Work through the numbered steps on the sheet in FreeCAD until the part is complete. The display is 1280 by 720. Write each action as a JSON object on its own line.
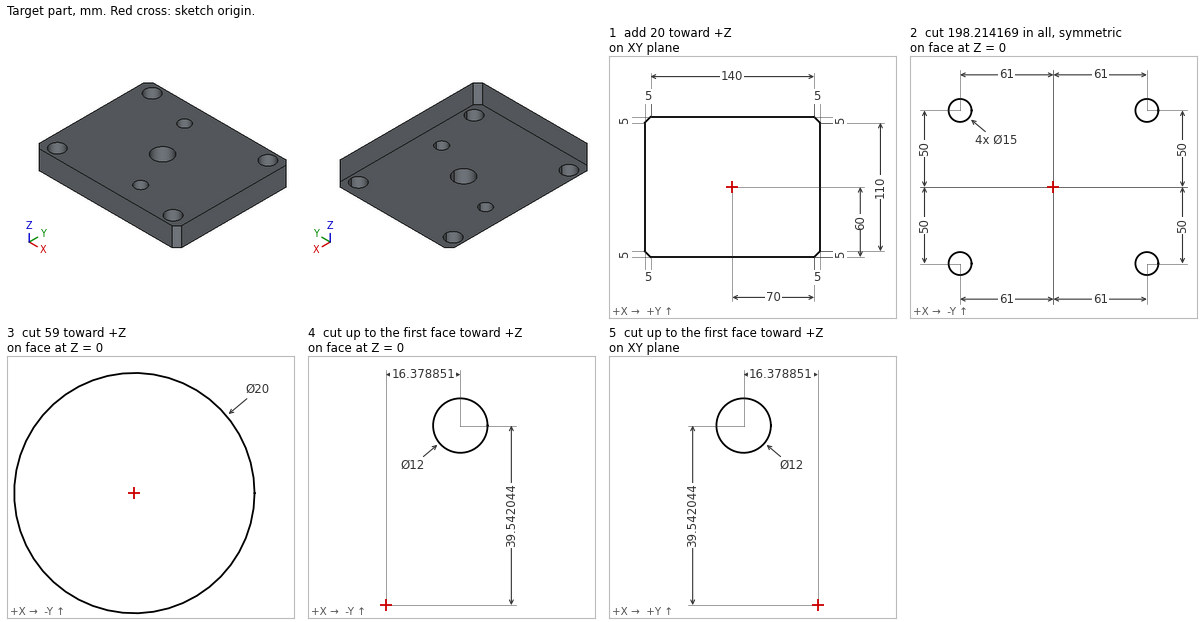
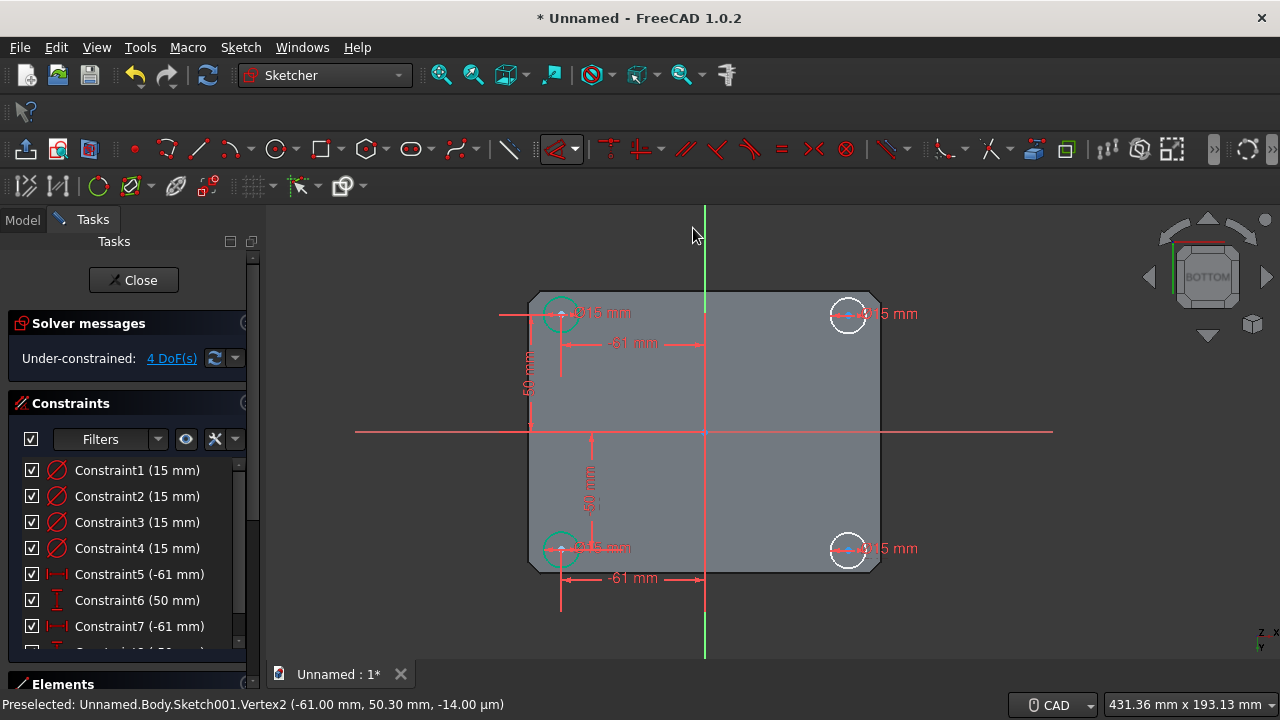
{"action": "left_click", "coordinate": [848, 316]}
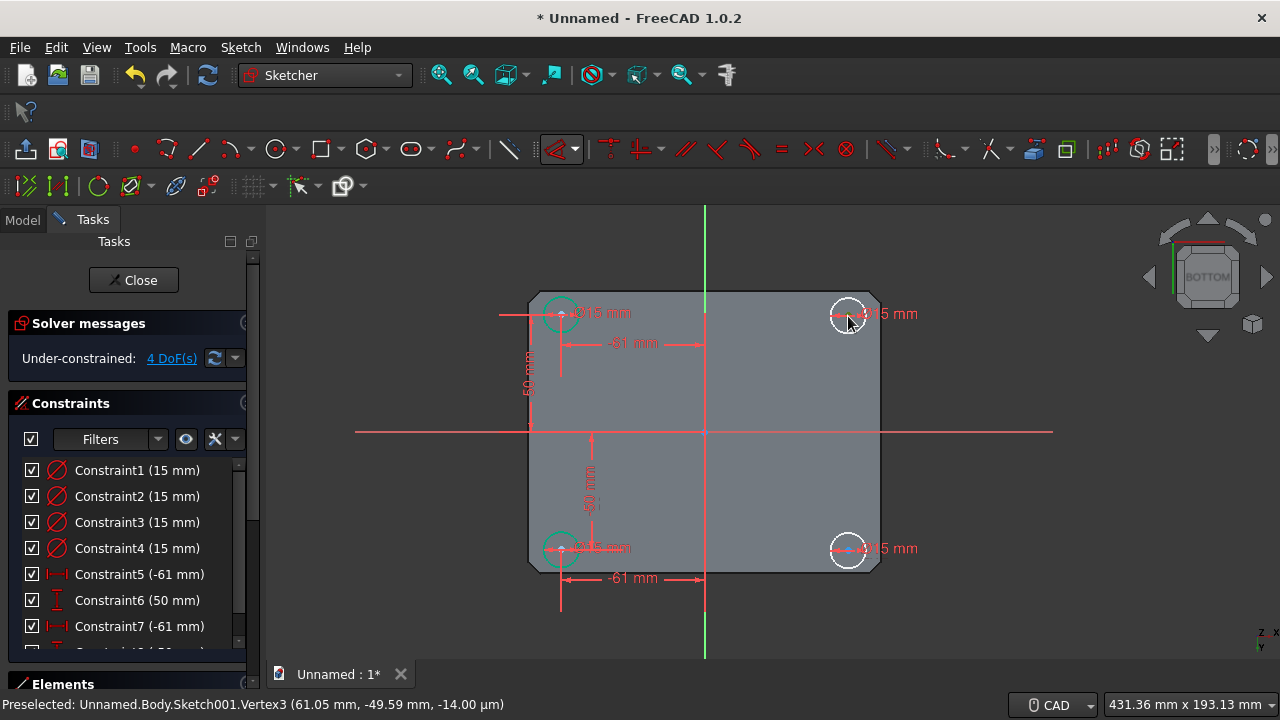
{"action": "key", "text": "l"}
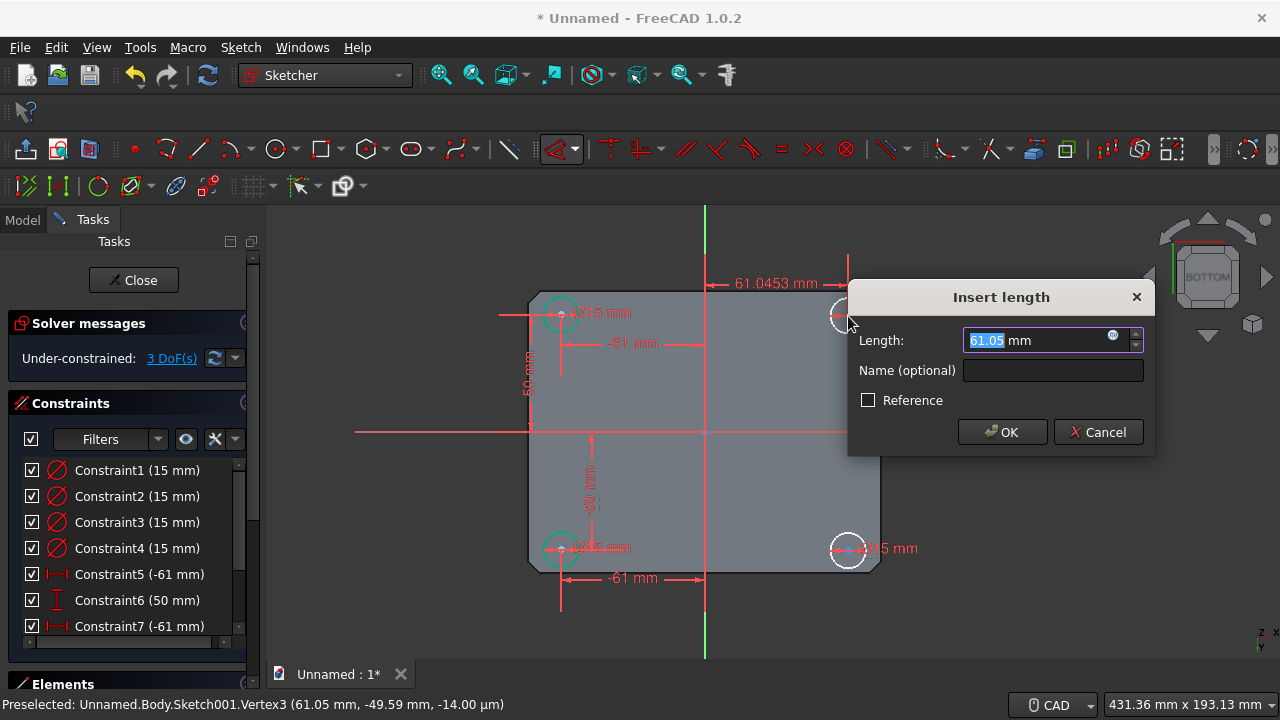
{"action": "type", "text": "61"}
{"action": "key", "text": "Return"}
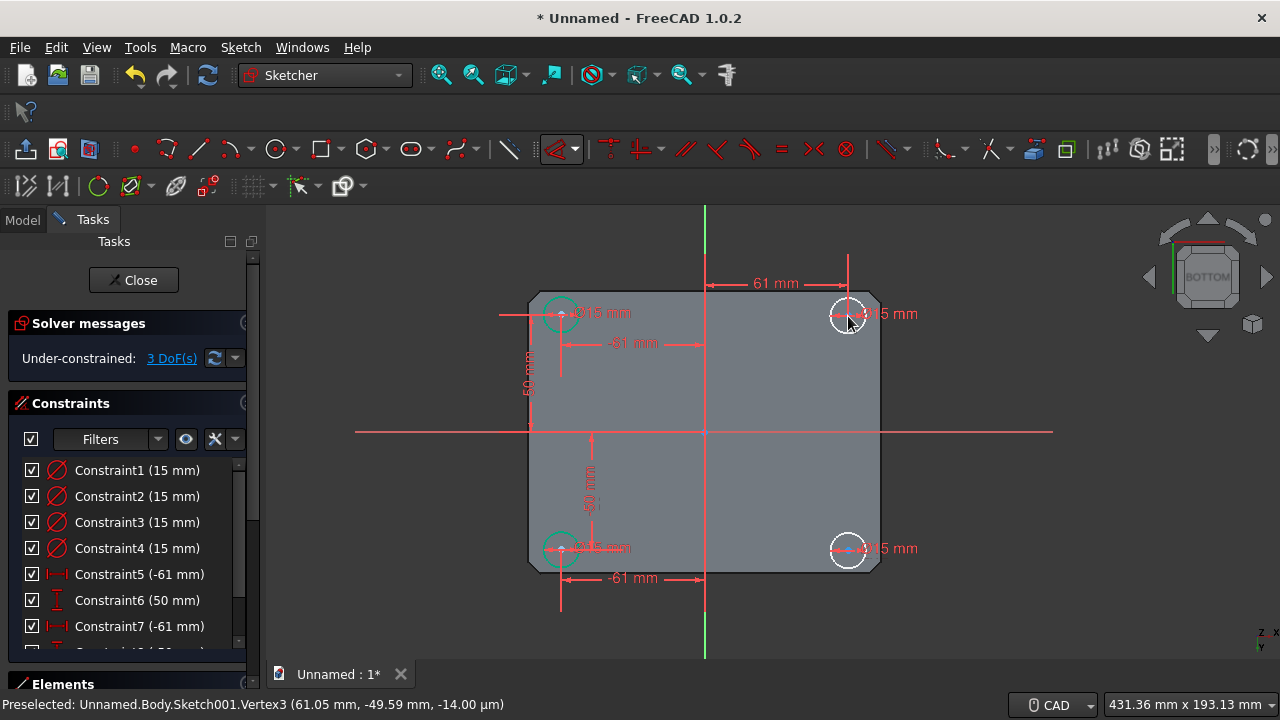
{"action": "left_click", "coordinate": [848, 316]}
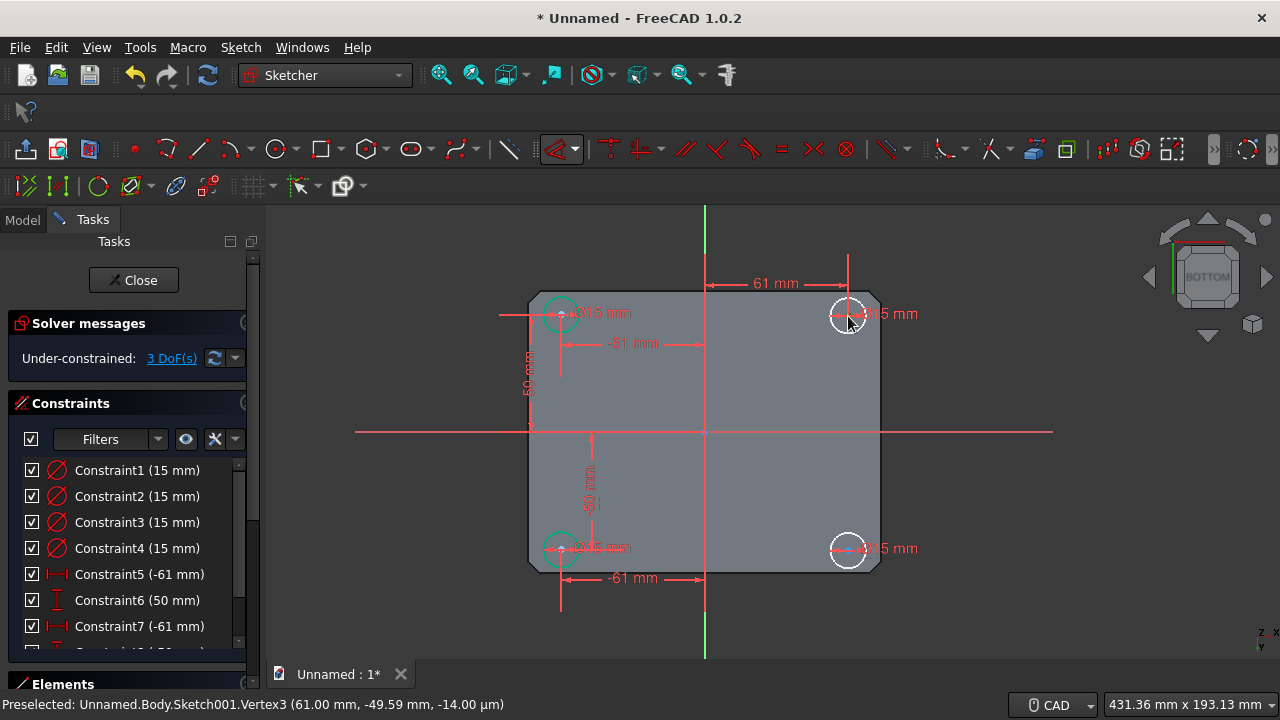
{"action": "left_click", "coordinate": [578, 150]}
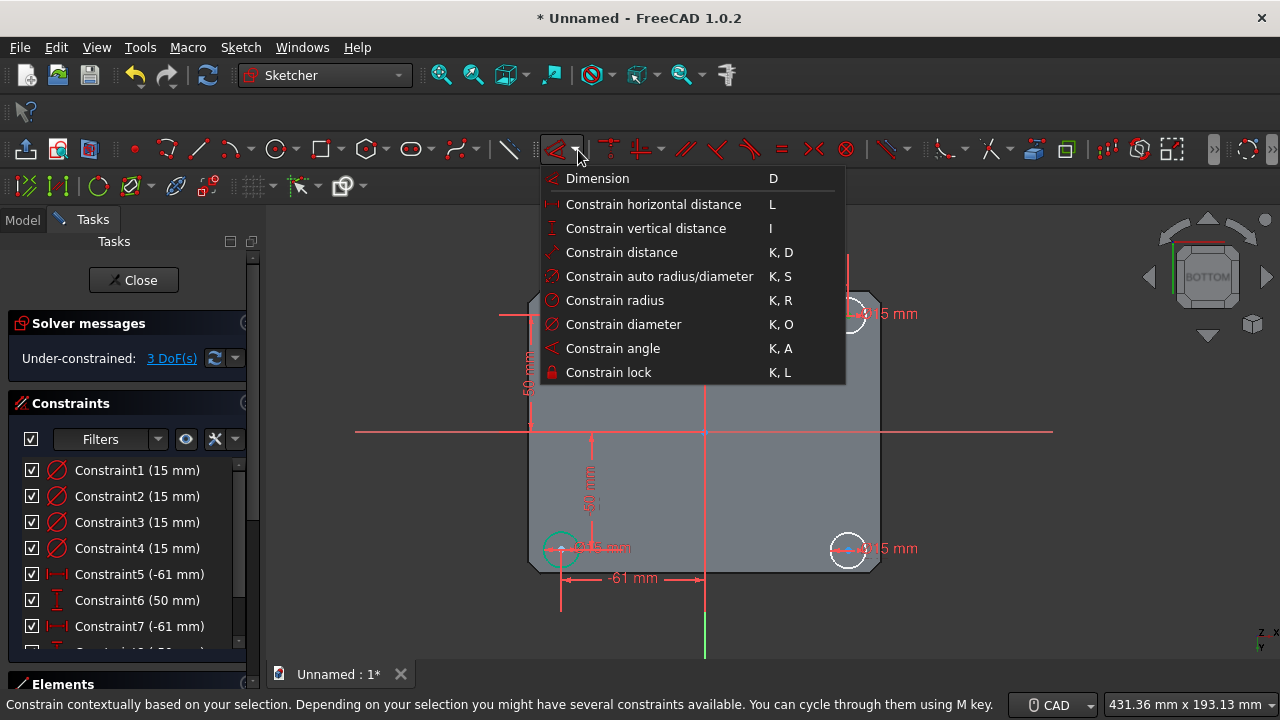
{"action": "left_click", "coordinate": [693, 228]}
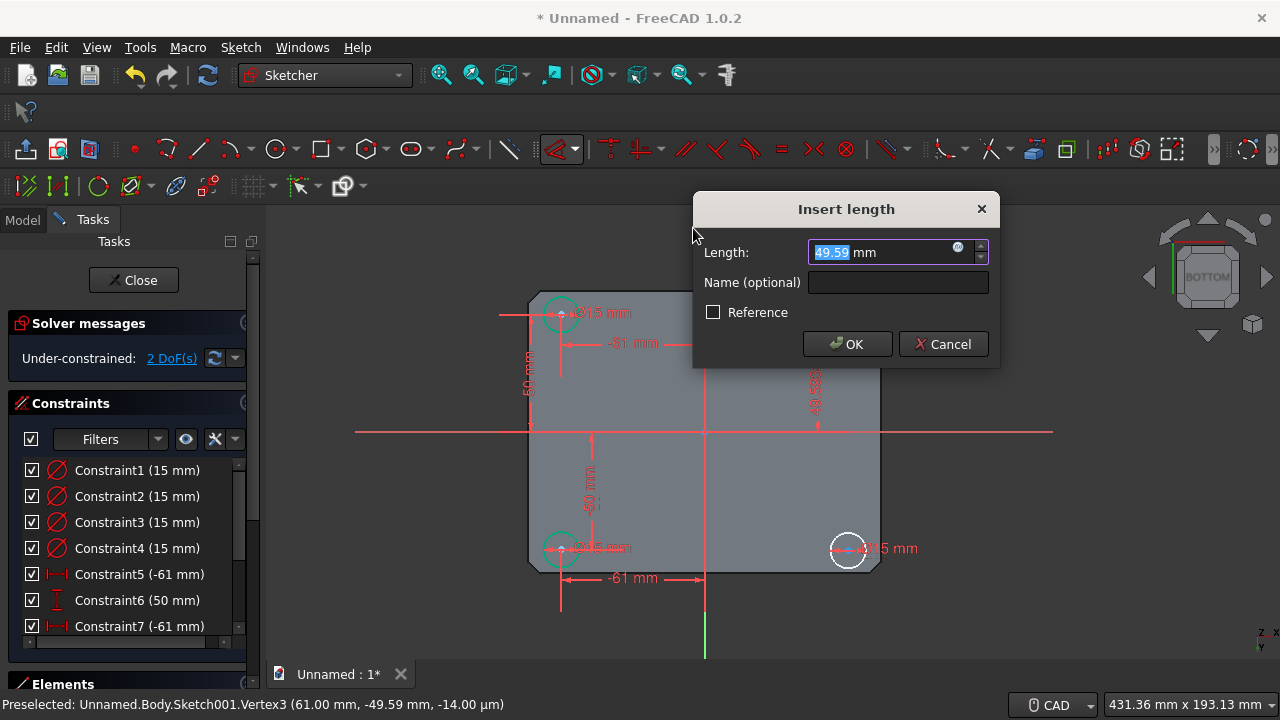
{"action": "type", "text": "50"}
{"action": "key", "text": "Return"}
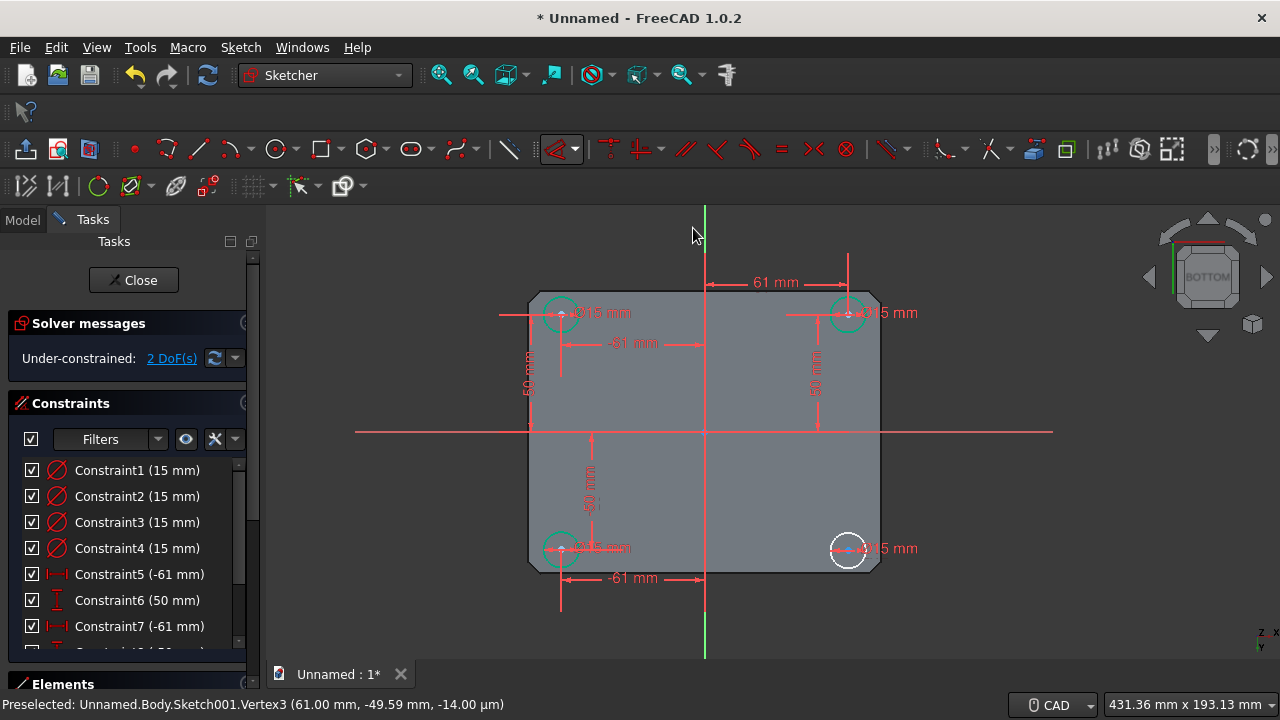
{"action": "left_click", "coordinate": [848, 551]}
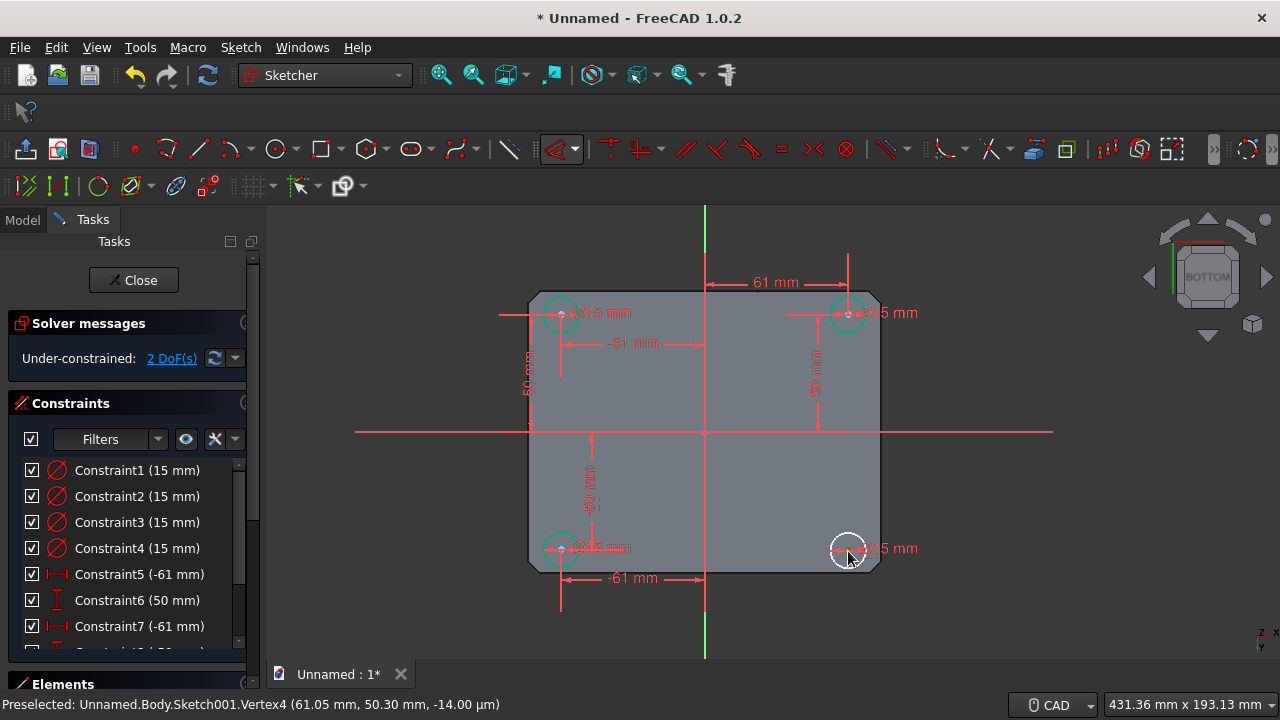
{"action": "key", "text": "l"}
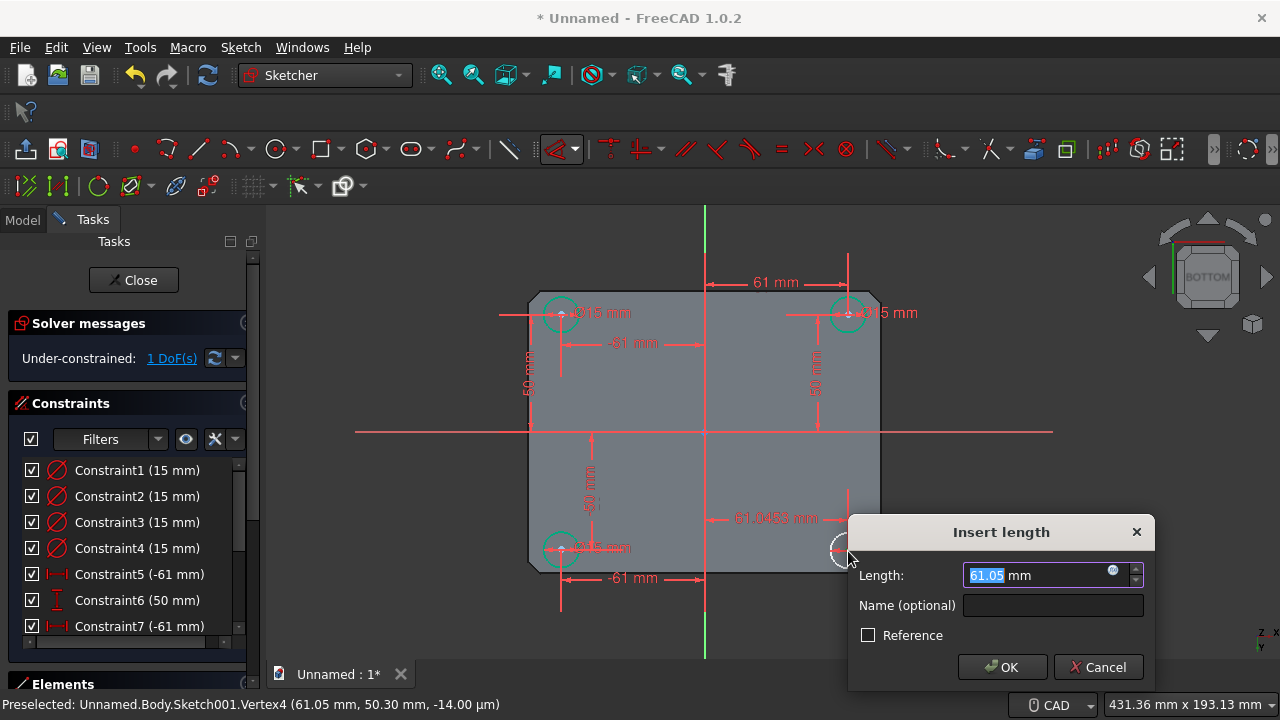
{"action": "type", "text": "61"}
{"action": "key", "text": "Return"}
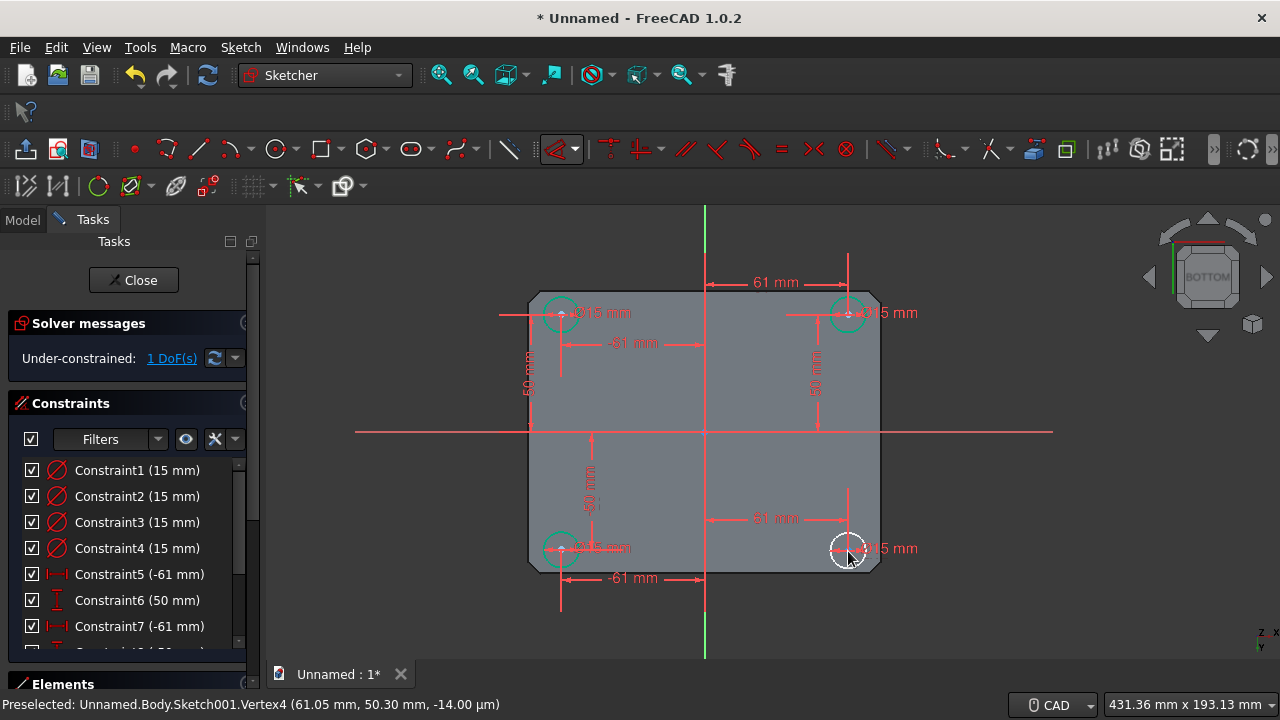
{"action": "left_click", "coordinate": [848, 551]}